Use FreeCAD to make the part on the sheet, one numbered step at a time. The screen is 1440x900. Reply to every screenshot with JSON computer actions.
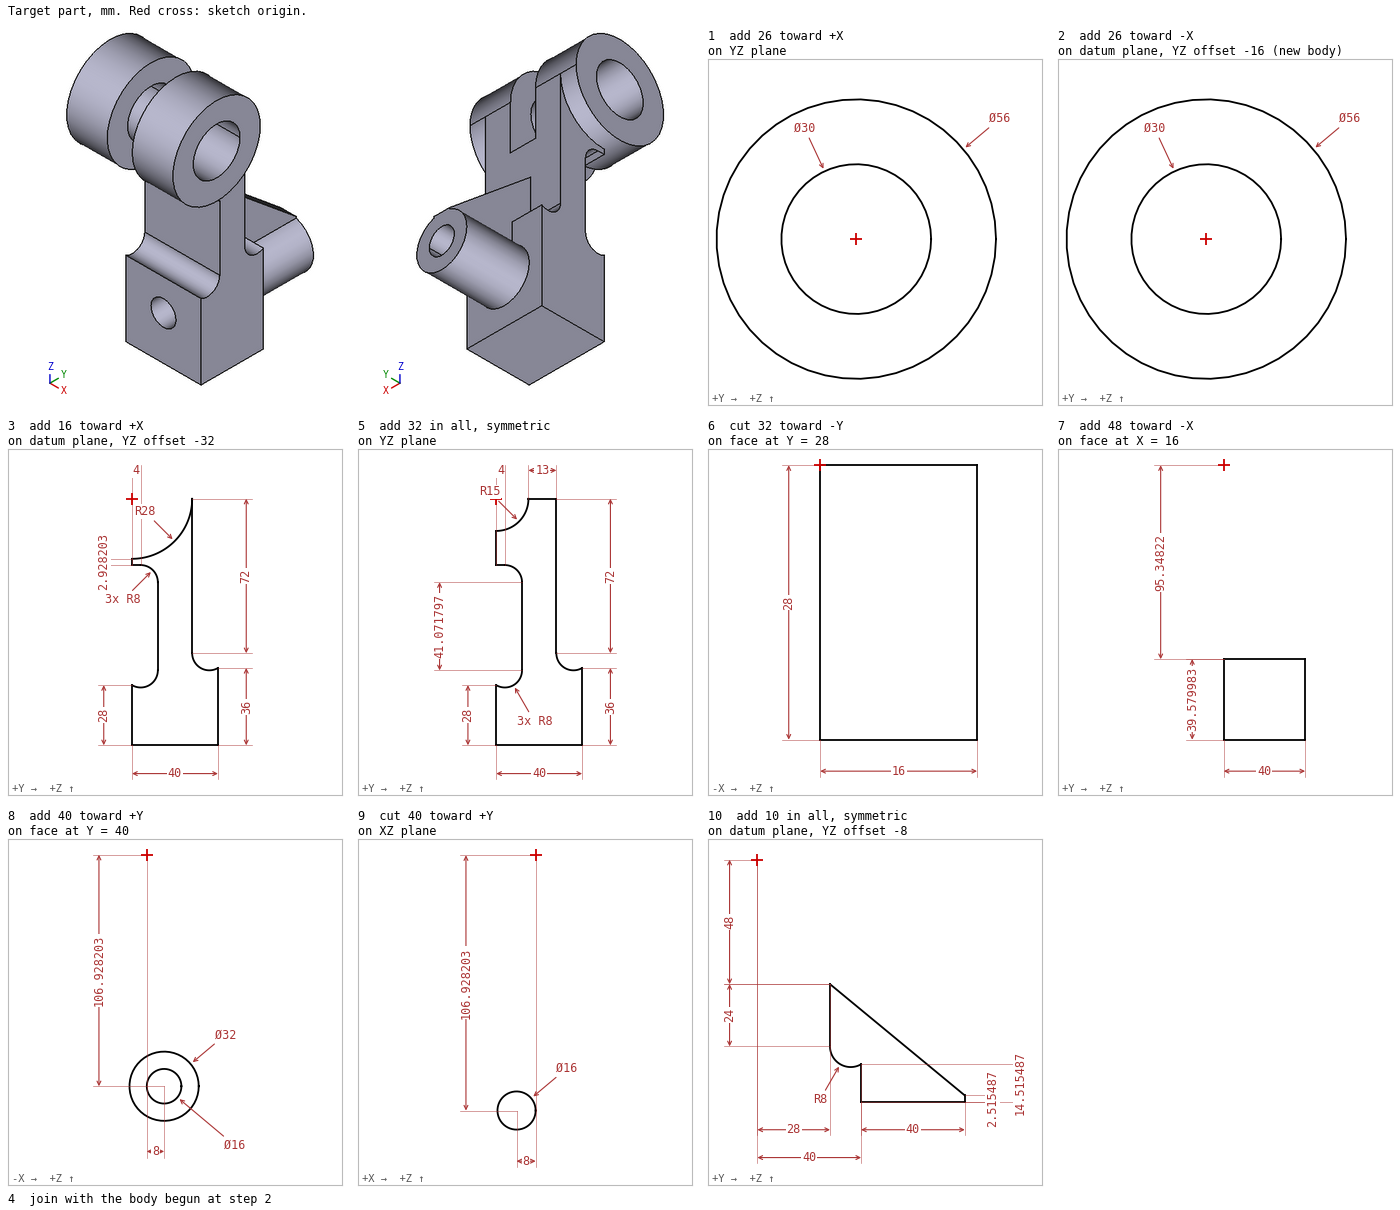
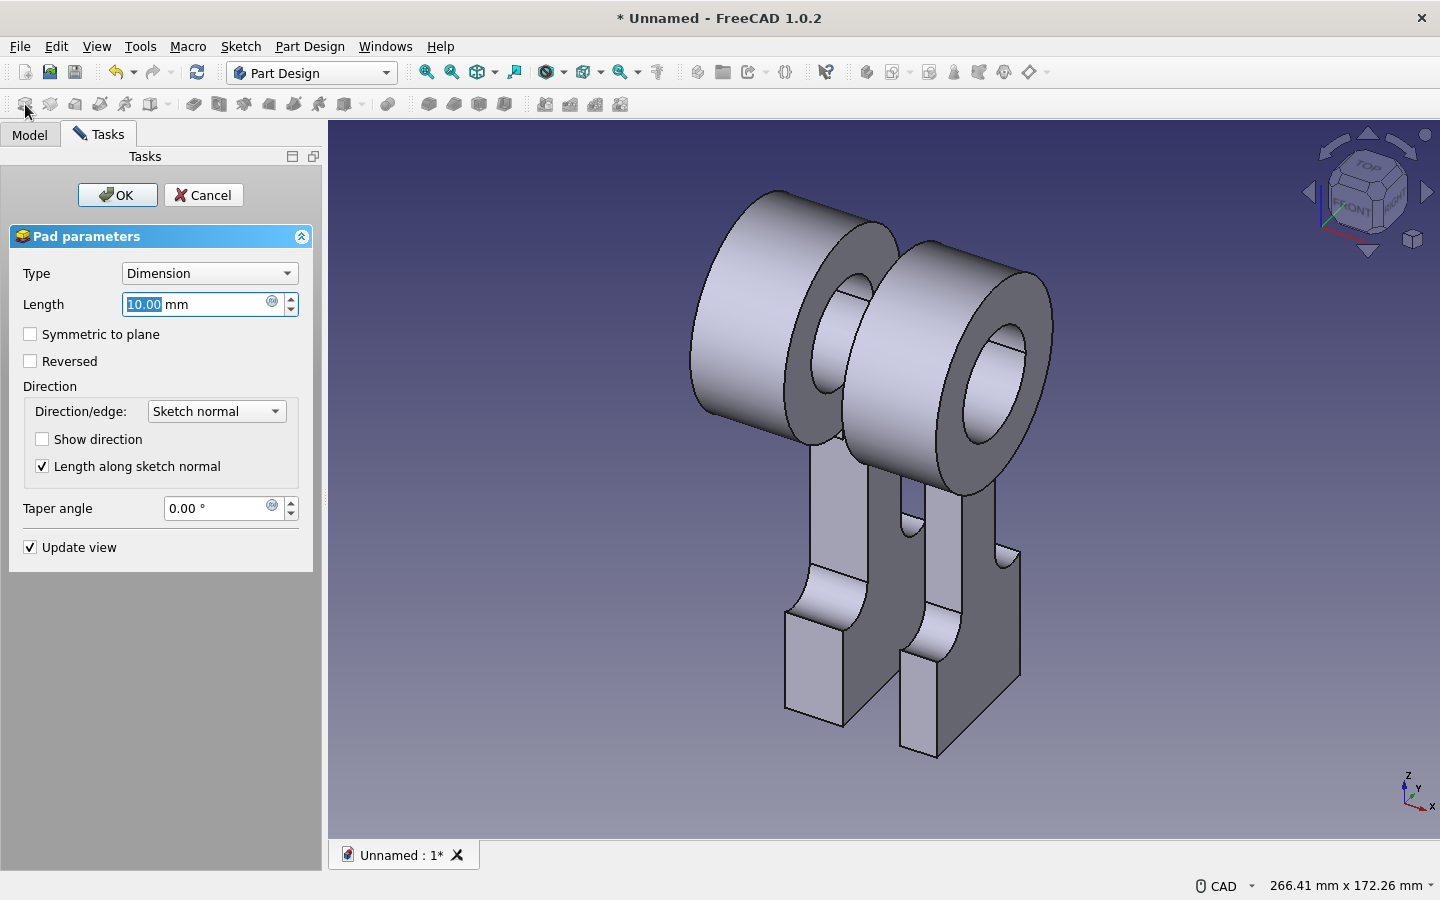
{"action": "type", "text": "32"}
{"action": "key", "text": "Tab"}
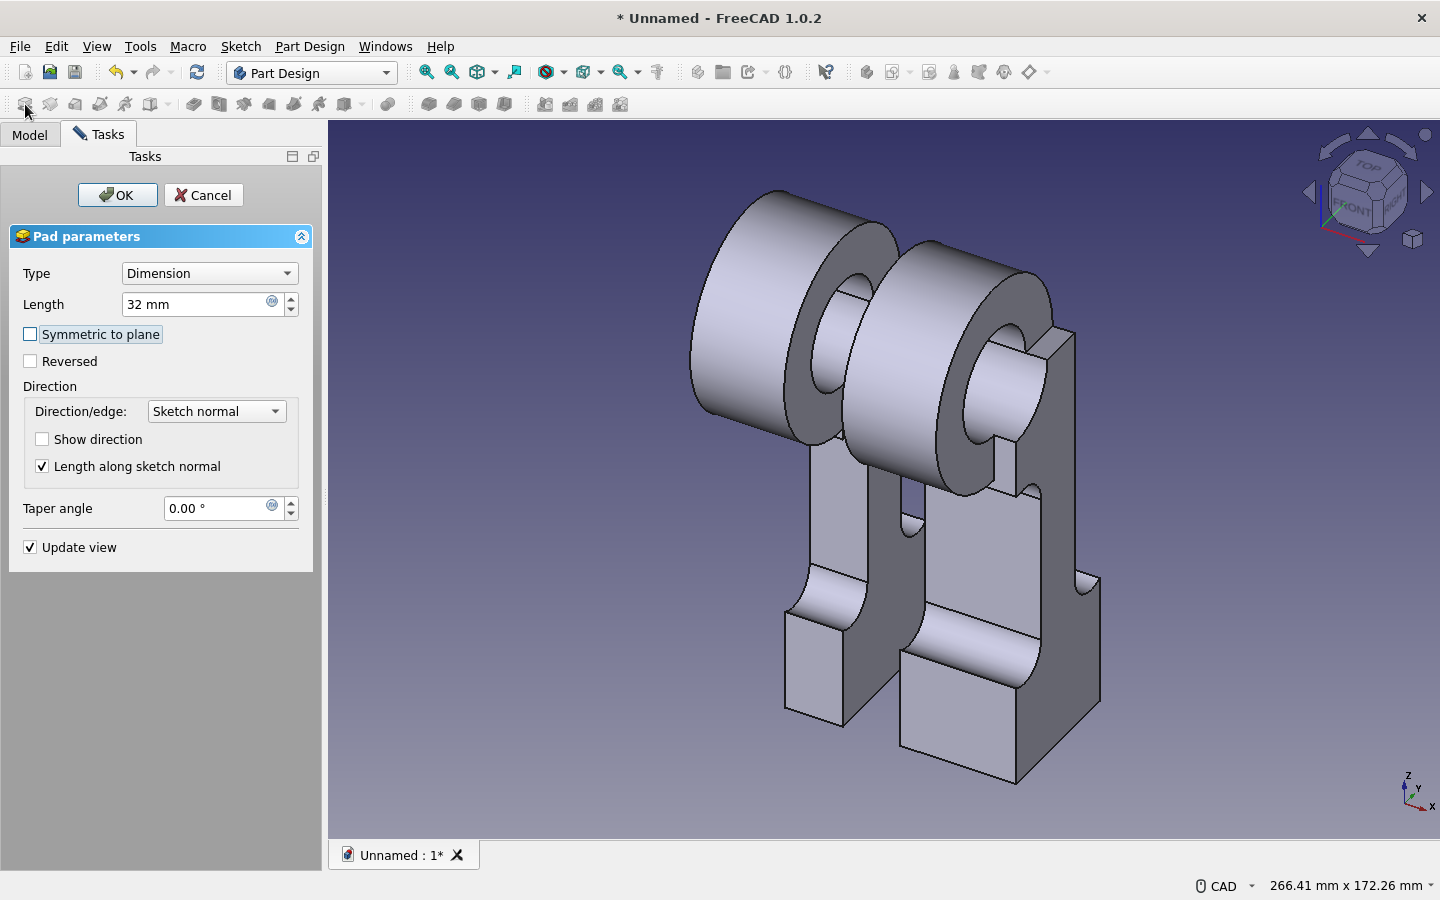
{"action": "left_click", "coordinate": [31, 334]}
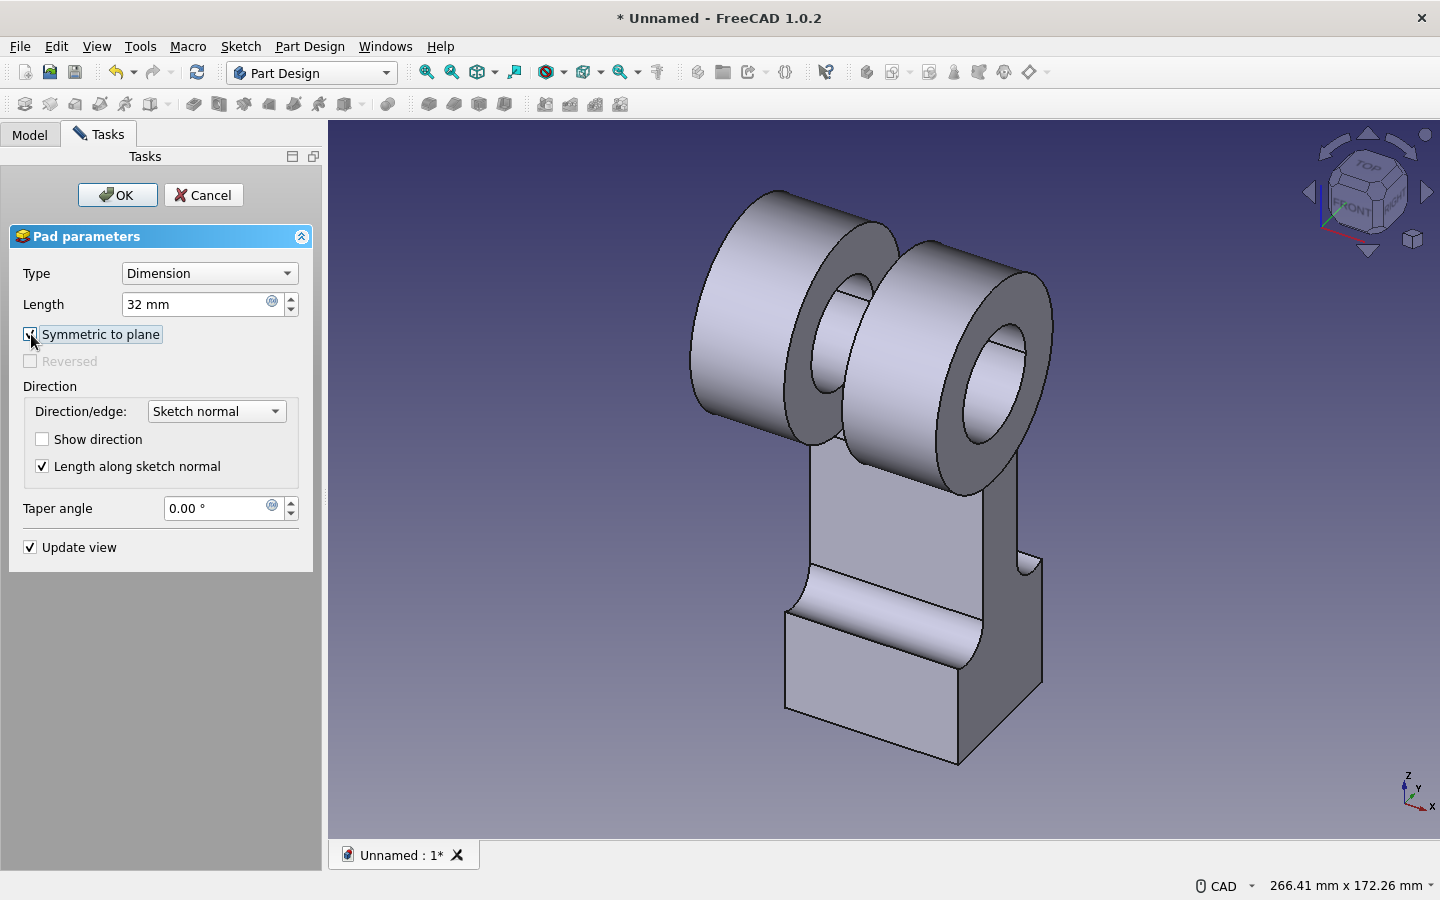
{"action": "left_click", "coordinate": [118, 195]}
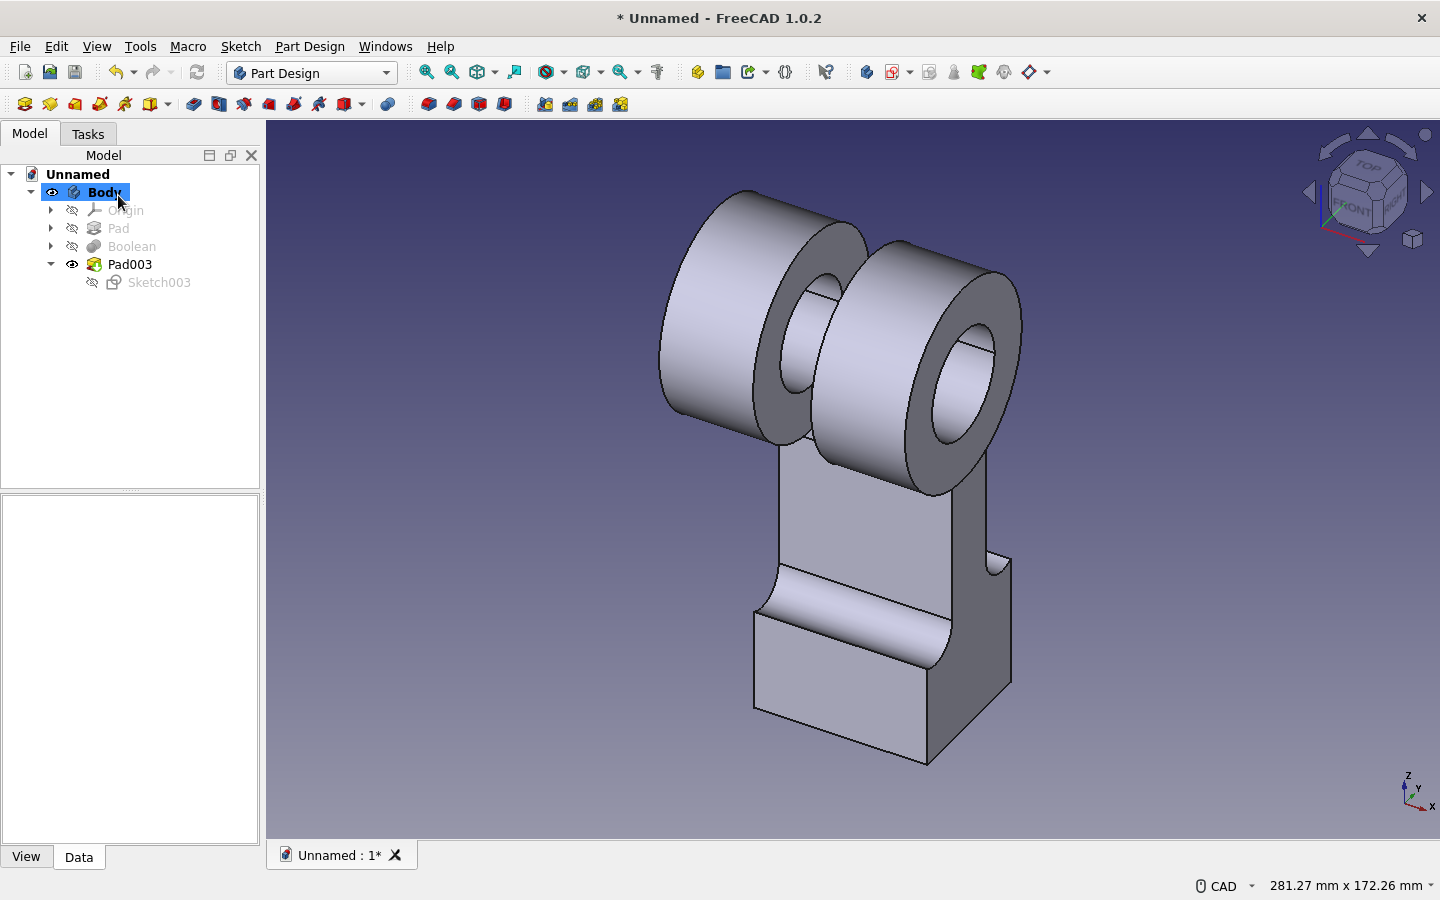
{"action": "key", "text": "4"}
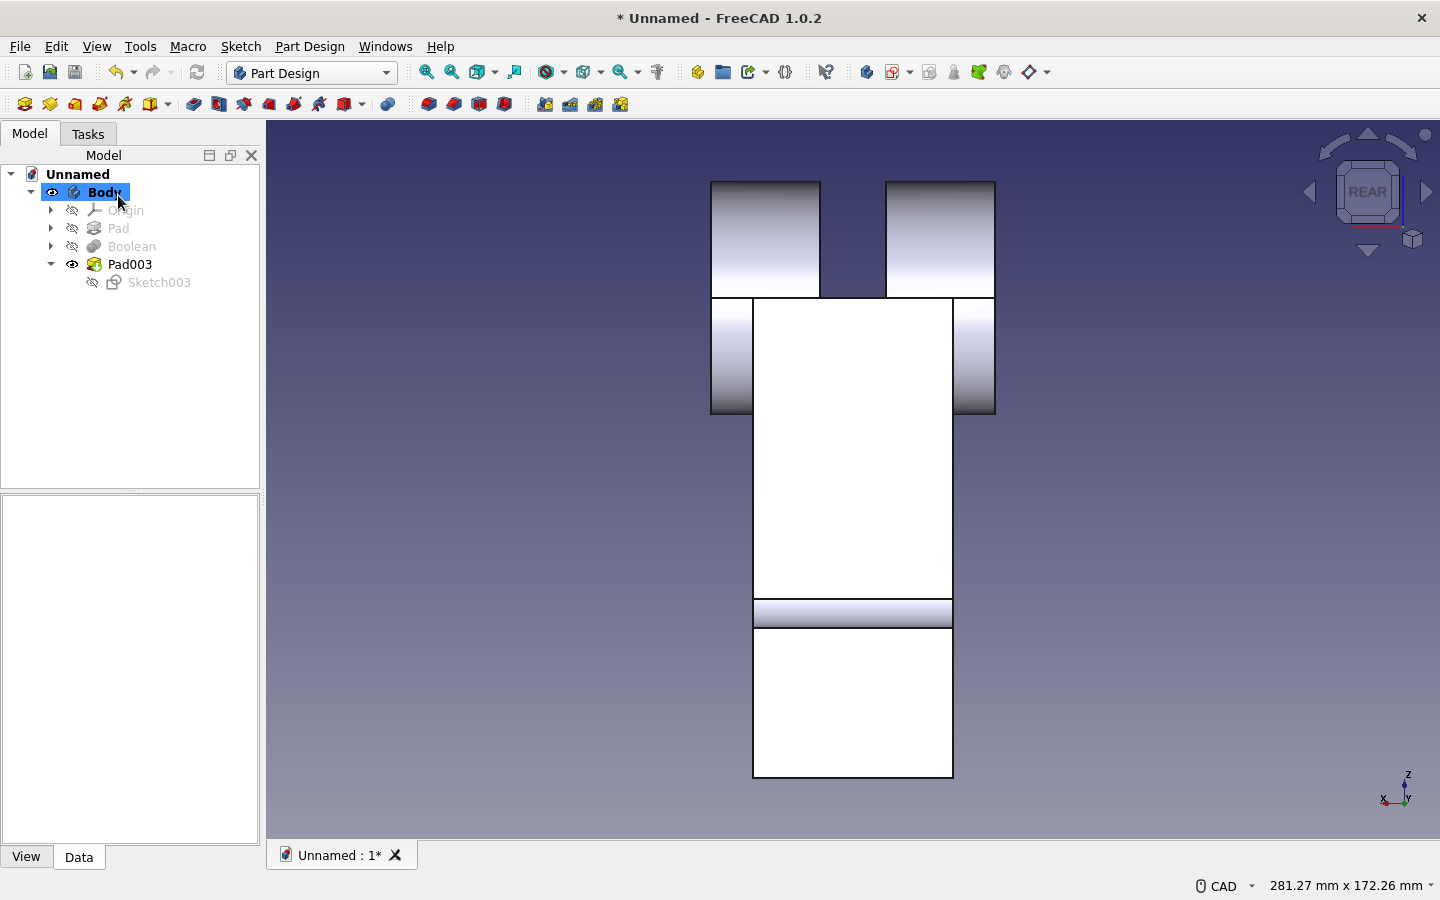
{"action": "left_click", "coordinate": [853, 404]}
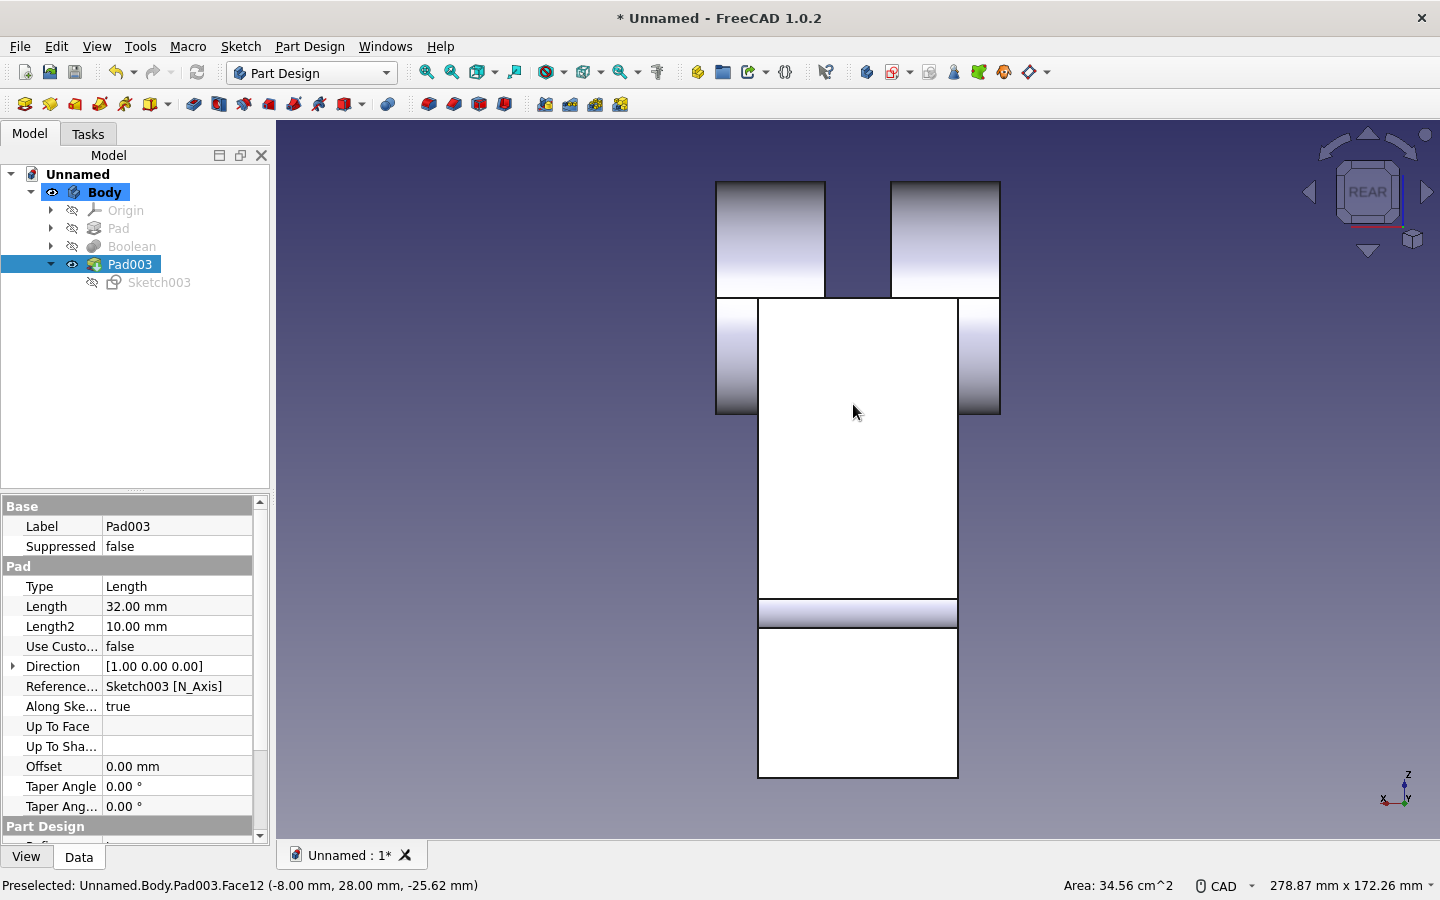
{"action": "left_click", "coordinate": [892, 72]}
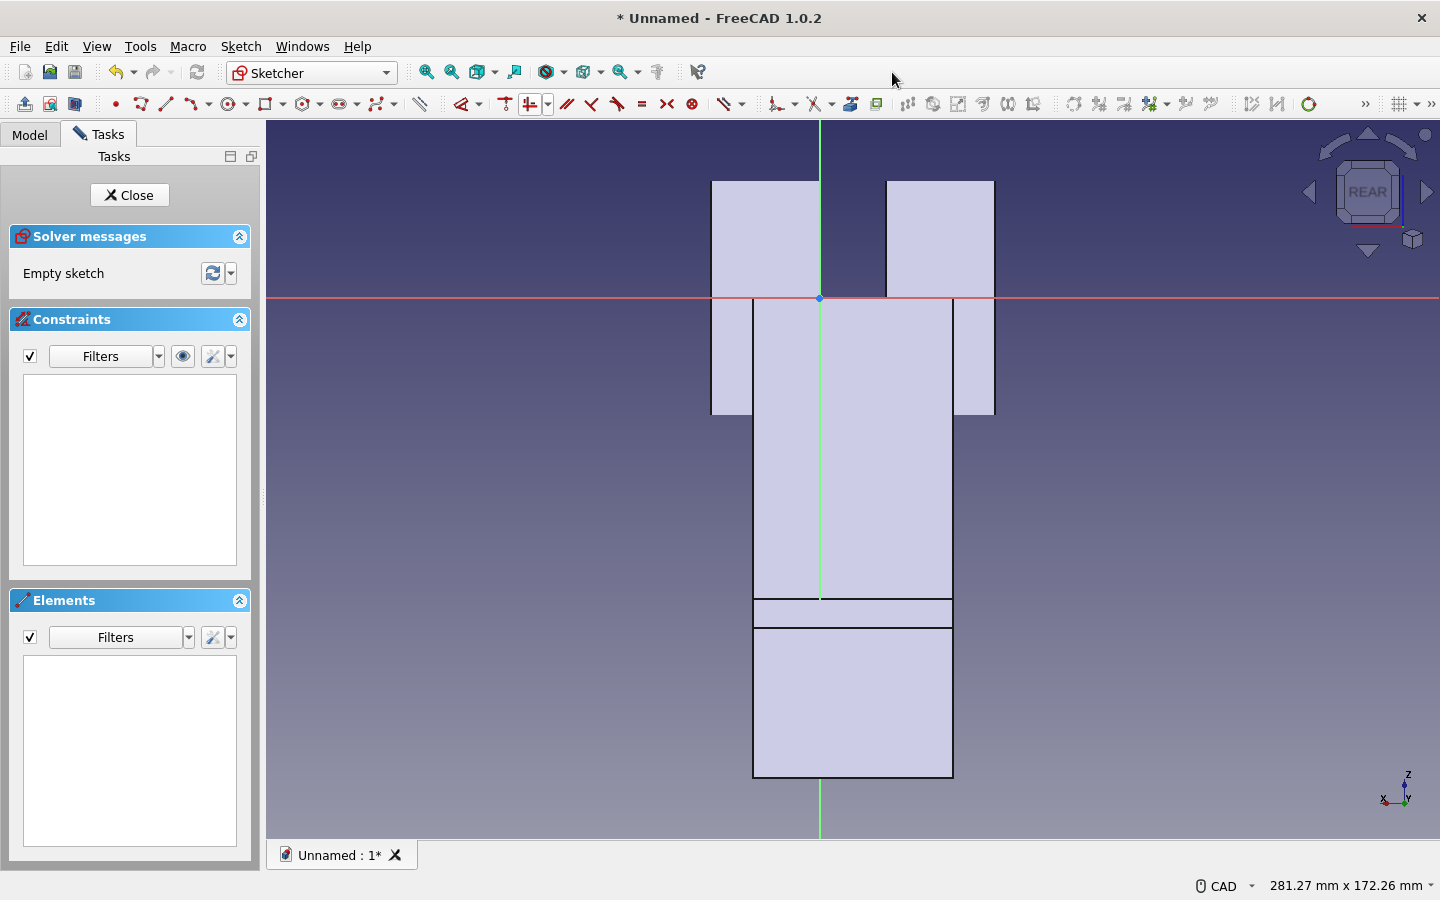
{"action": "scroll", "coordinate": [875, 316], "scroll_direction": "up", "scroll_amount": 7}